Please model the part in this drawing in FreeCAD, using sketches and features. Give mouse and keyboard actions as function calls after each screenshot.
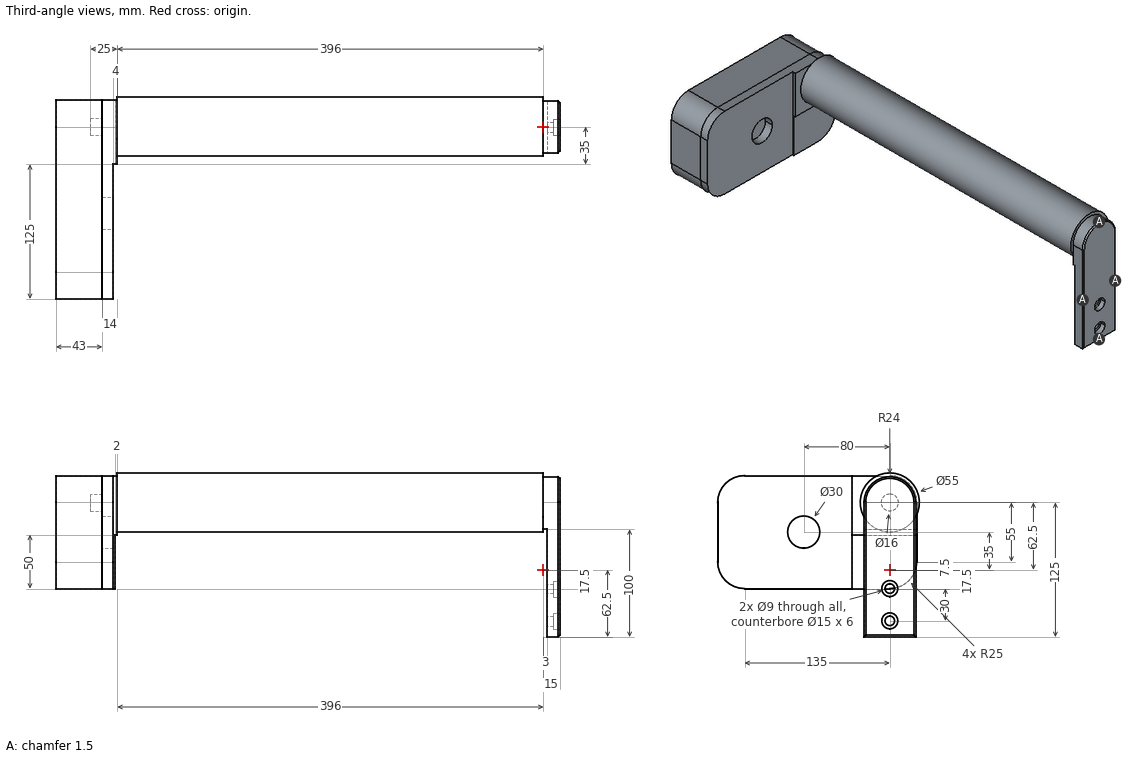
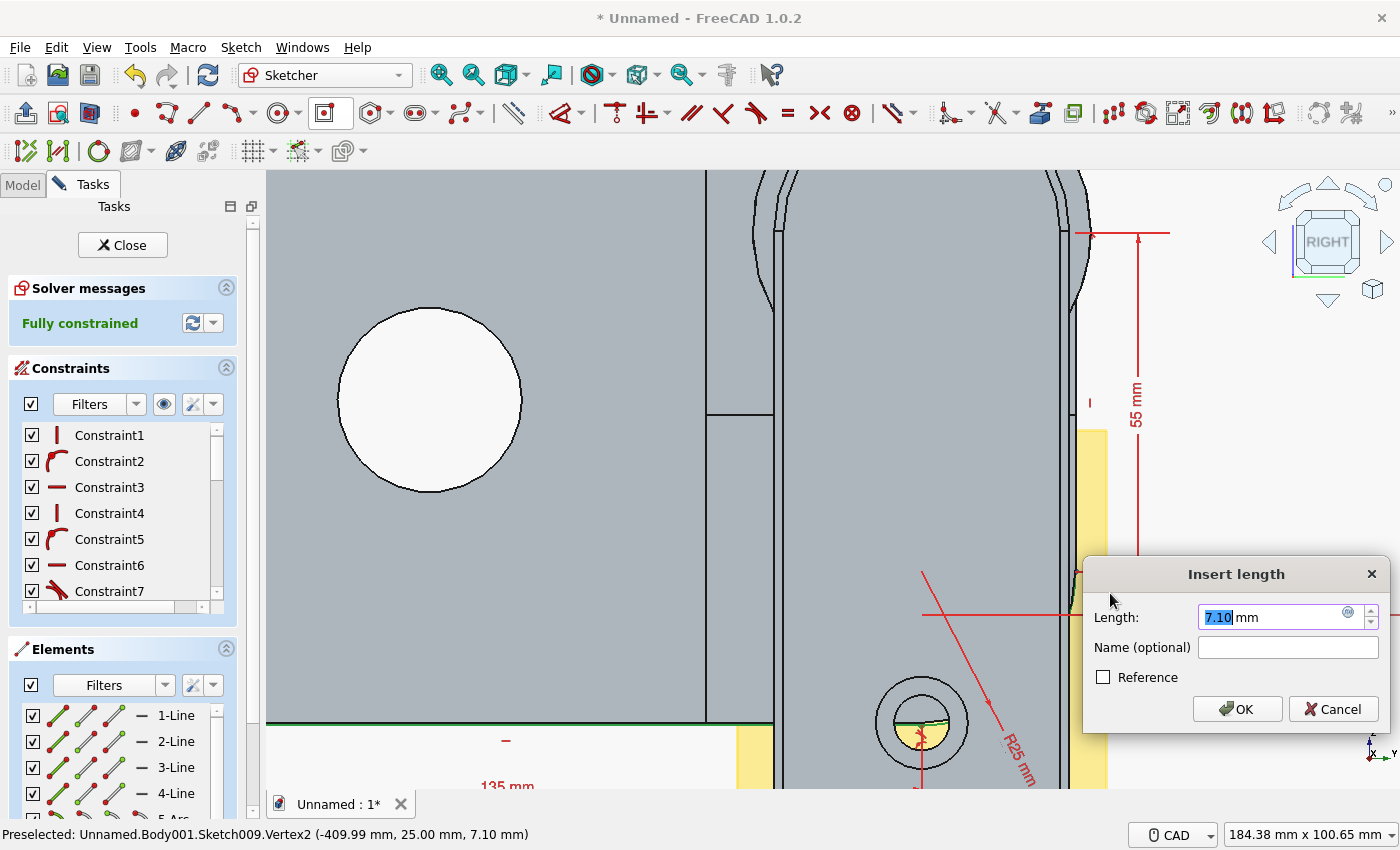
text(7.5)
key(Return)
key(Escape)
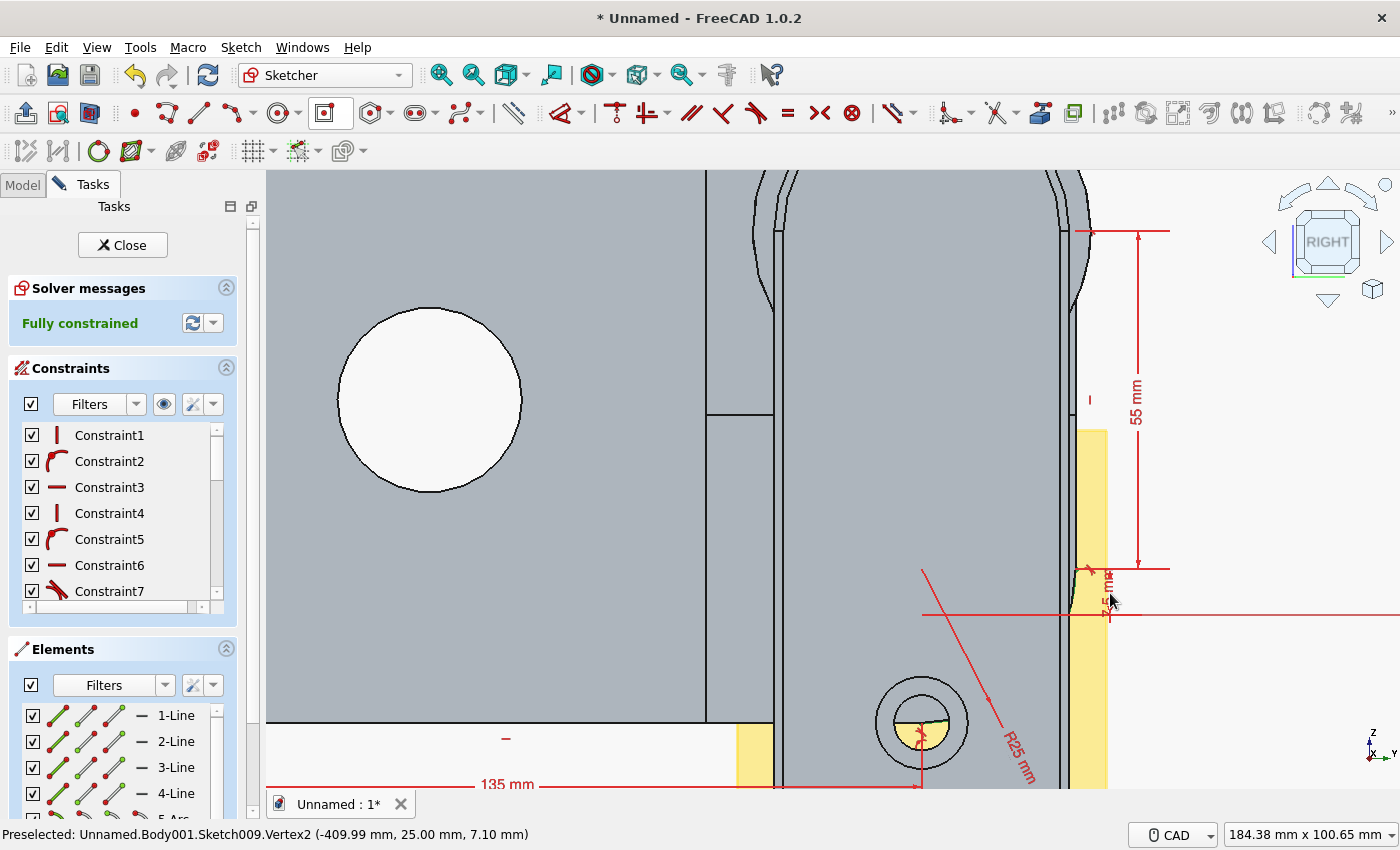
click(123, 245)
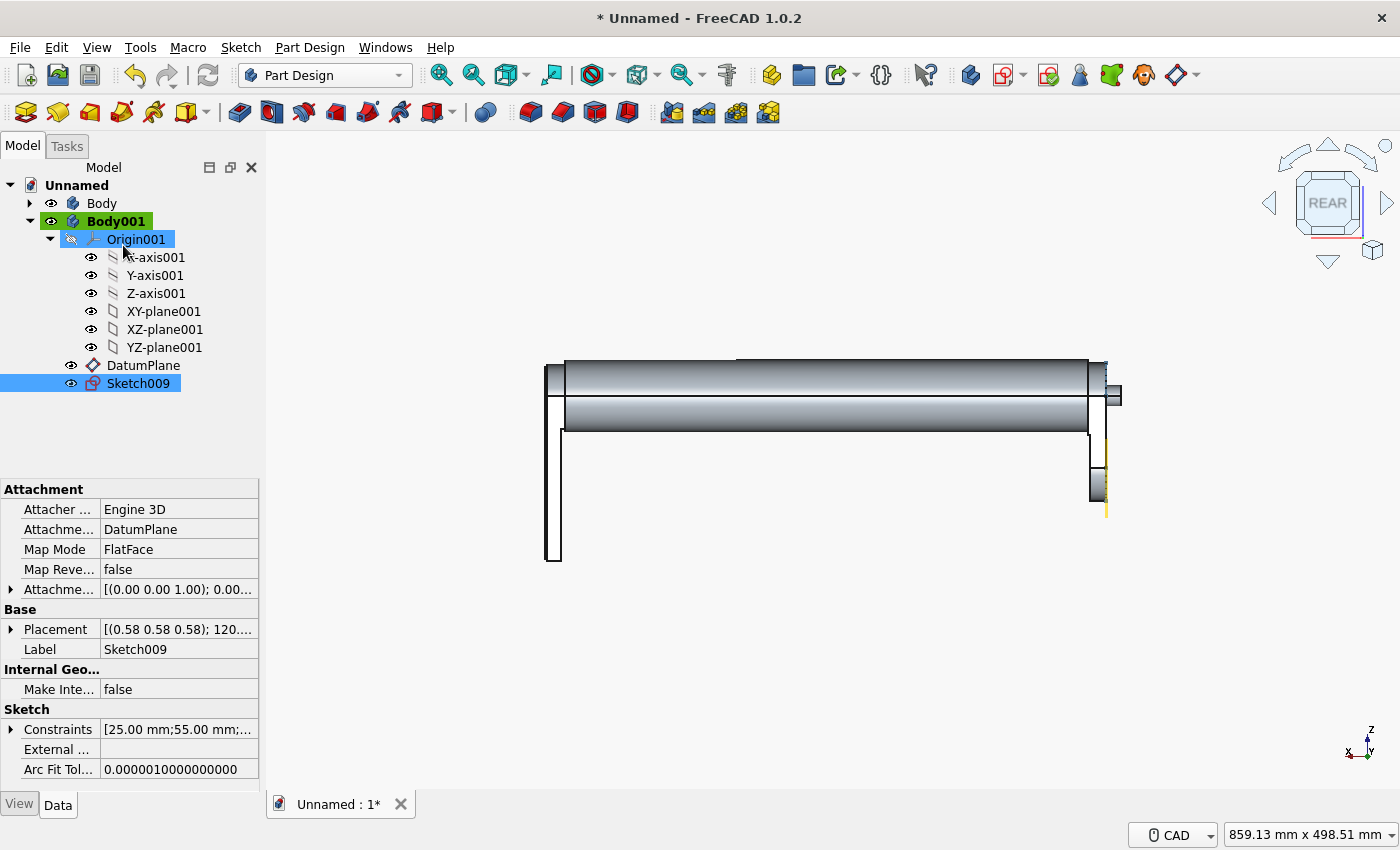
click(26, 112)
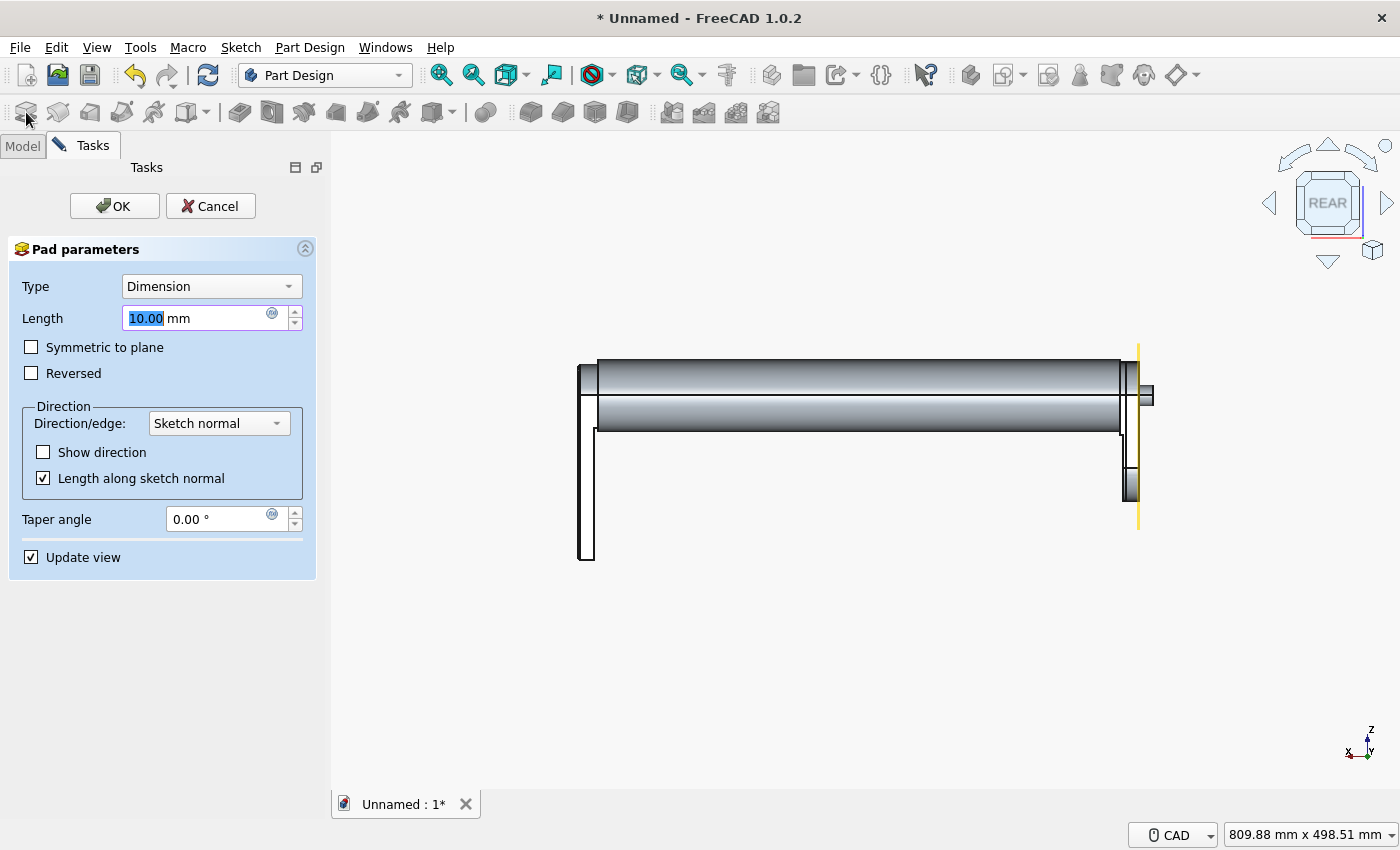
text(43)
key(Tab)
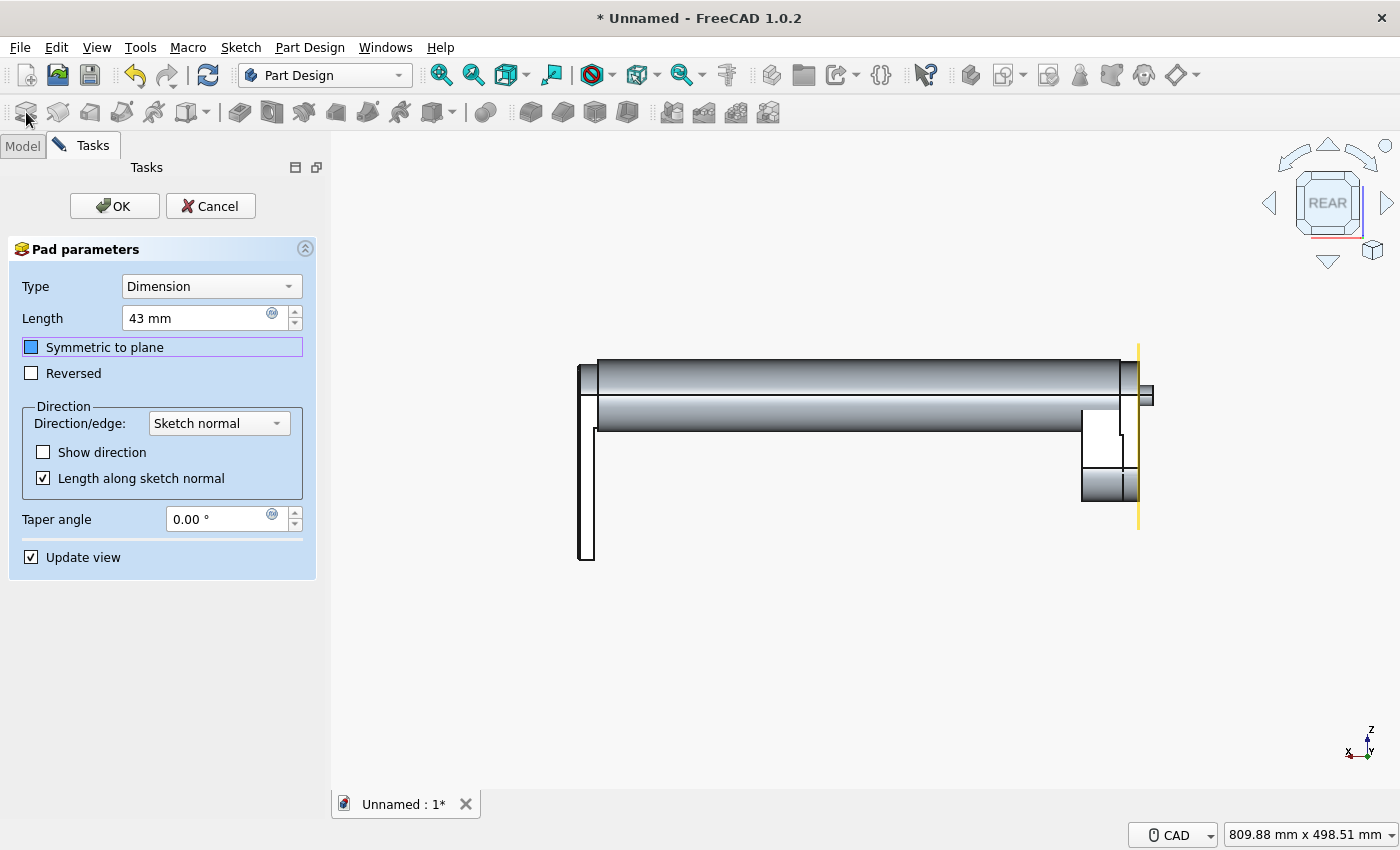
click(30, 373)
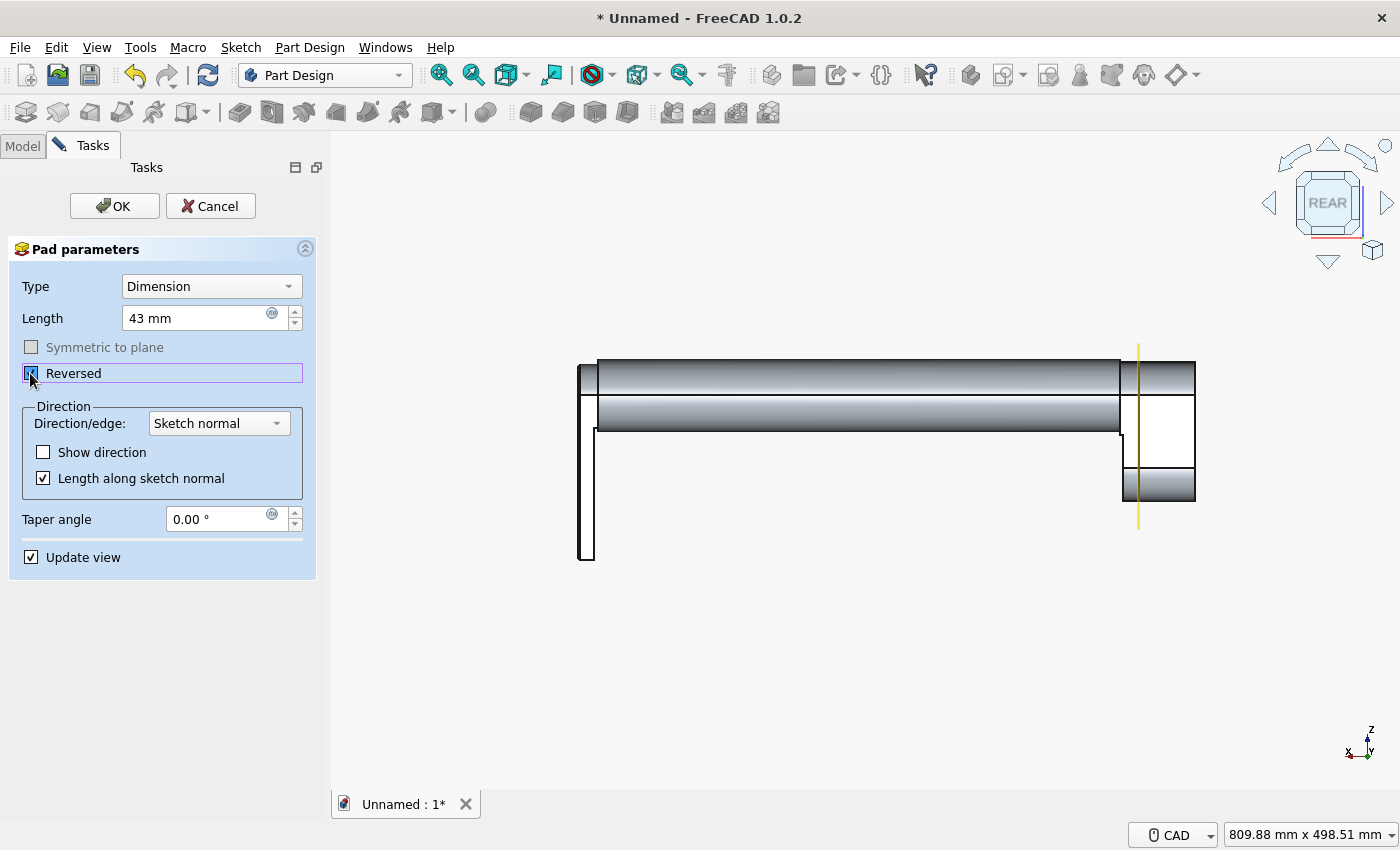
click(115, 206)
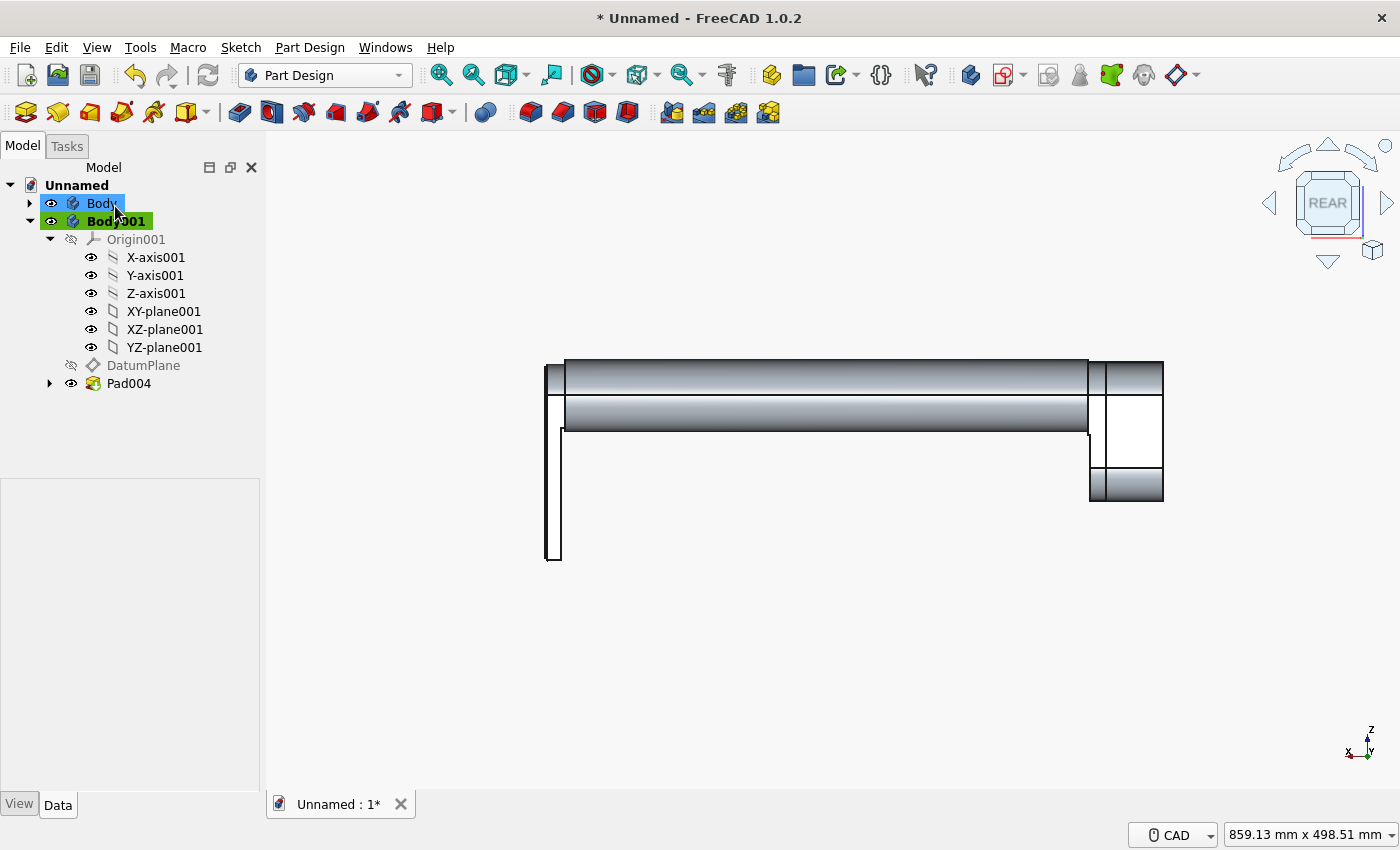
key(0)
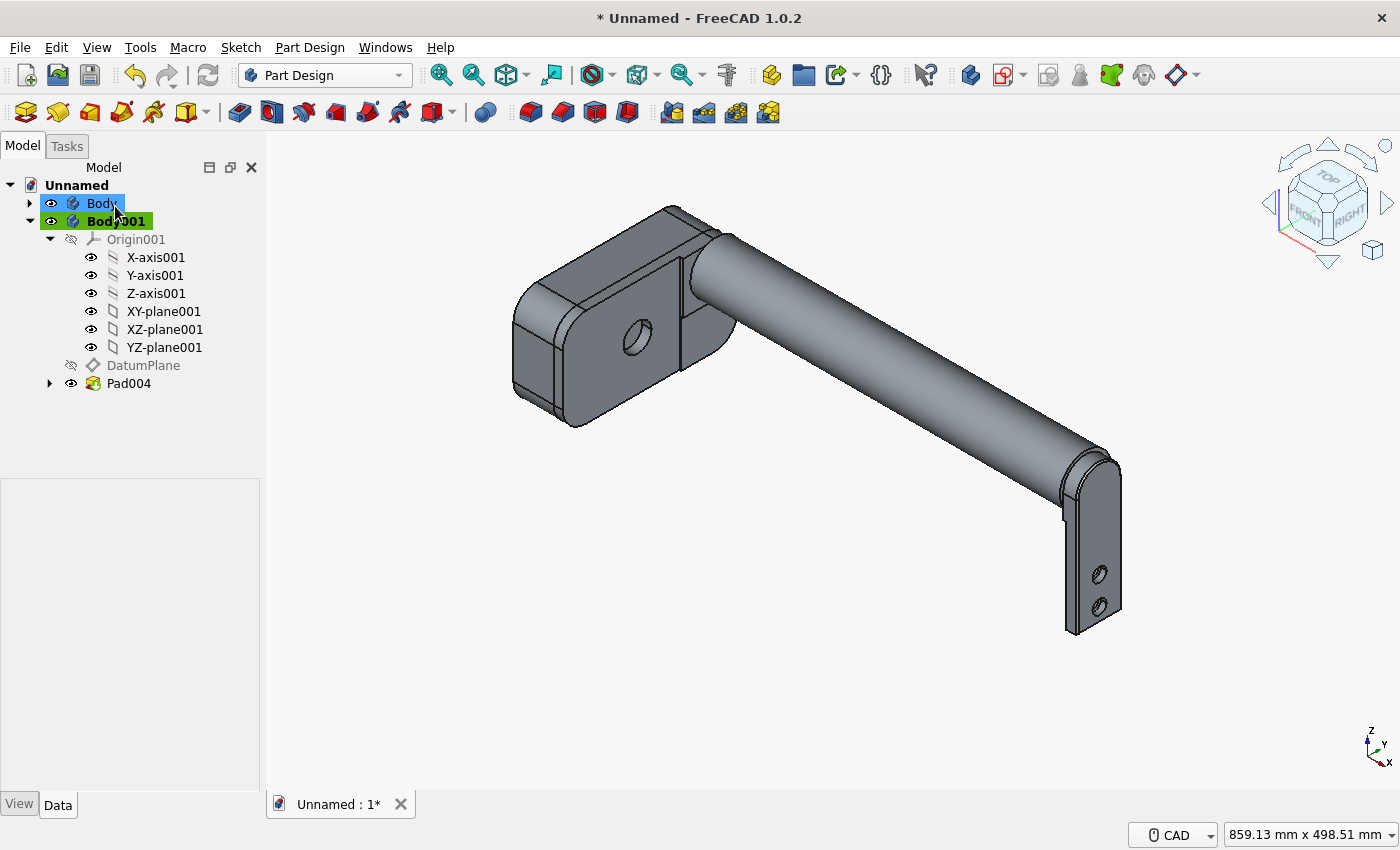
click(442, 76)